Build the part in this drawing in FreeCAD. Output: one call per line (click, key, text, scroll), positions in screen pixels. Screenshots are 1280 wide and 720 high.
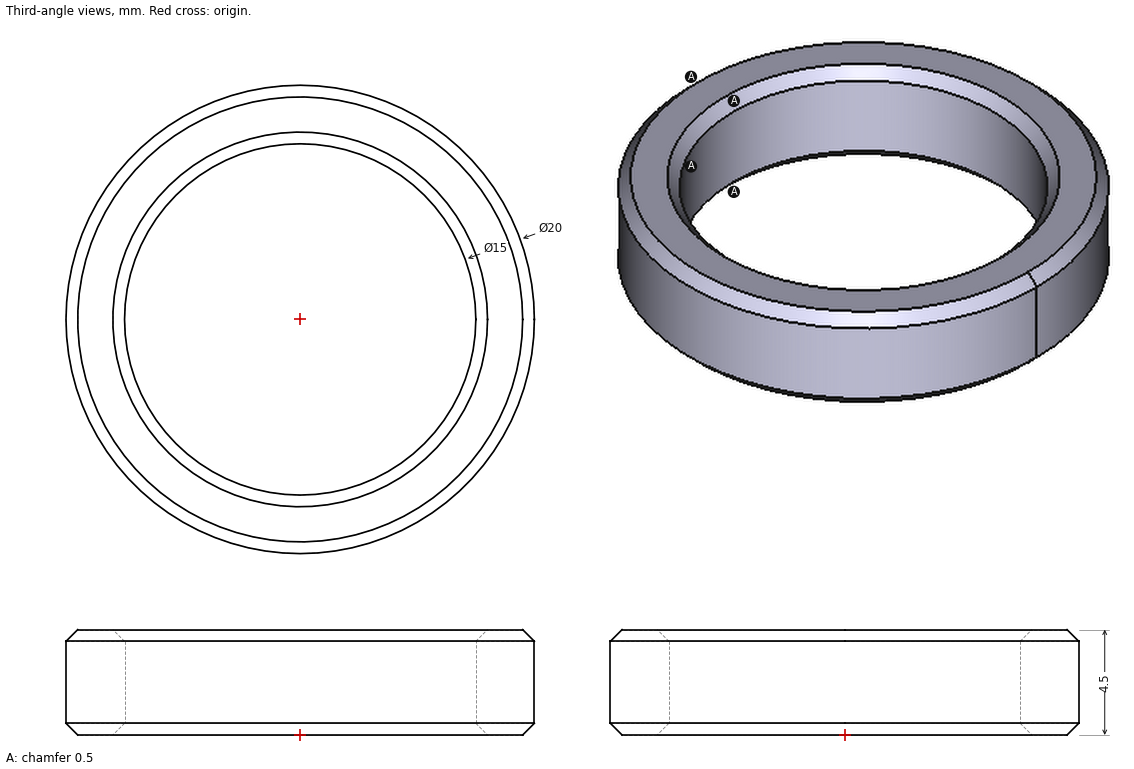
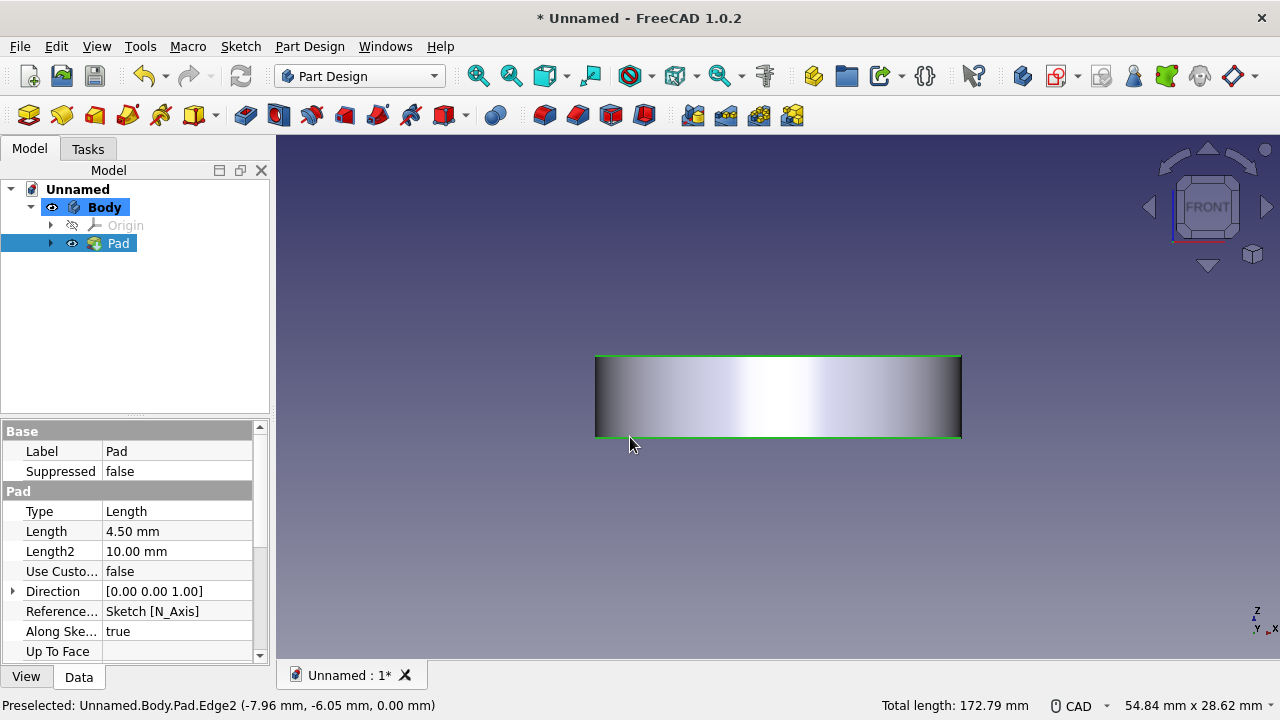
key(3)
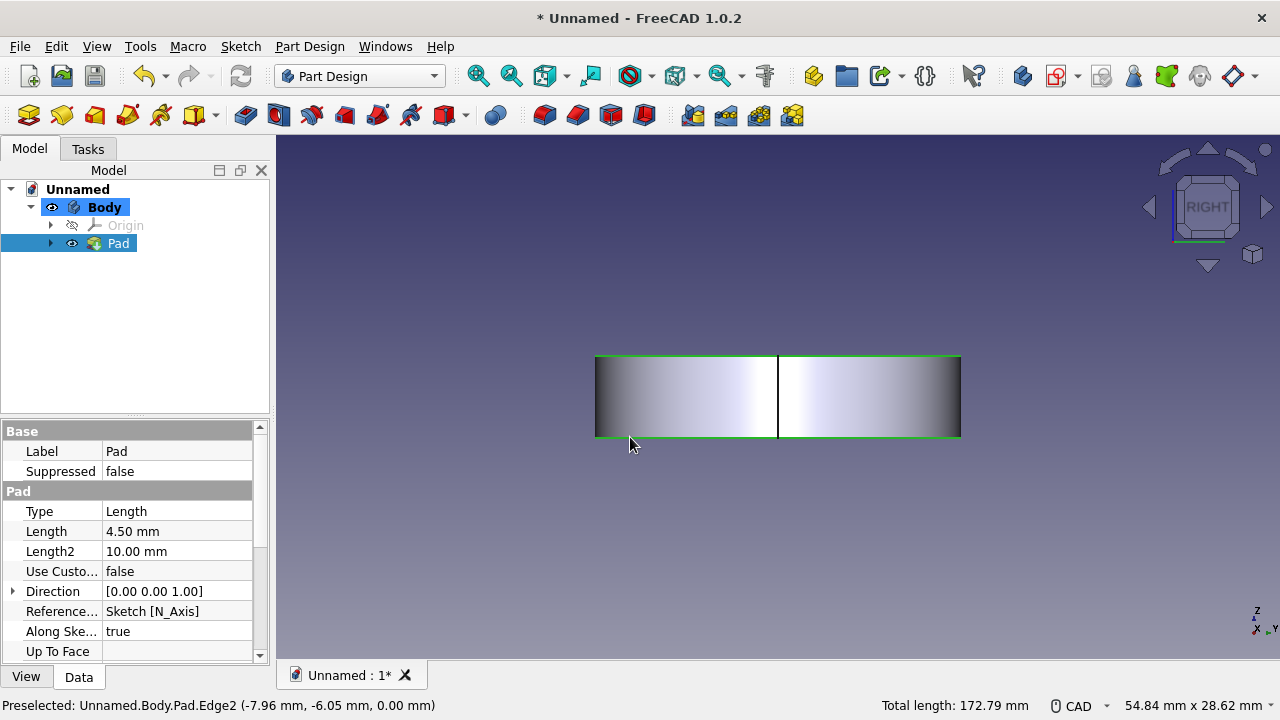
click(479, 76)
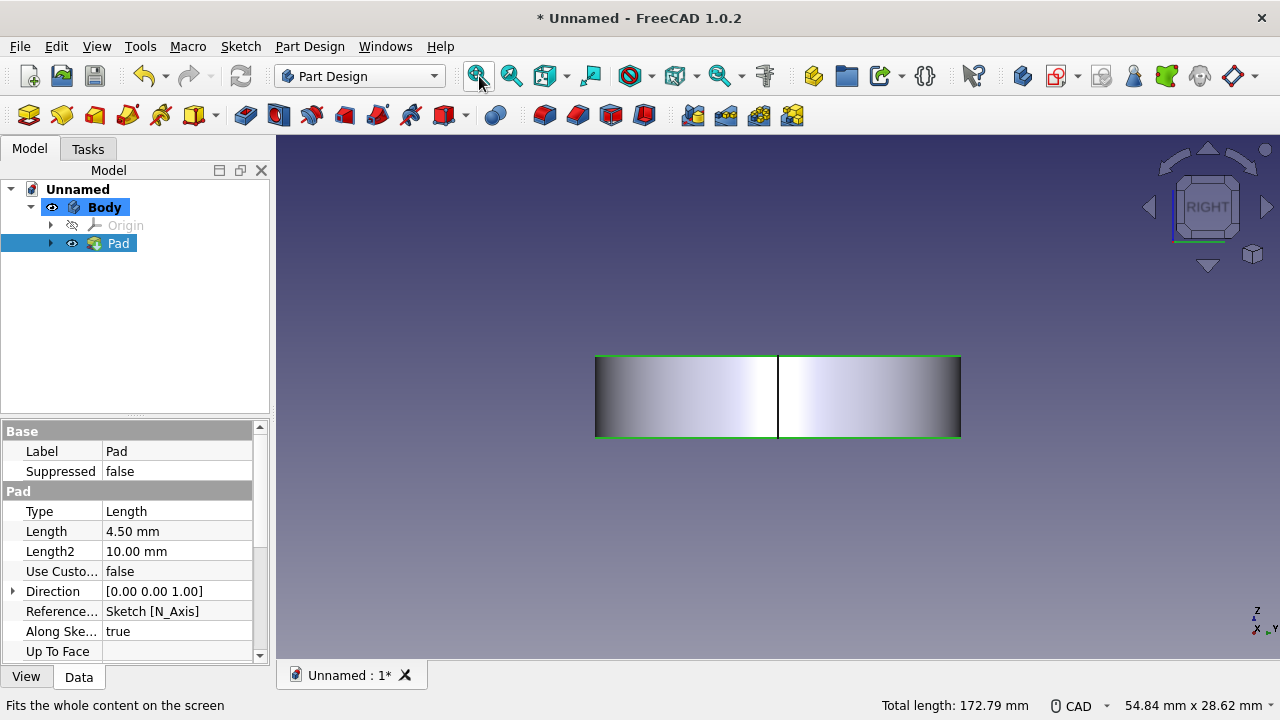
key(5)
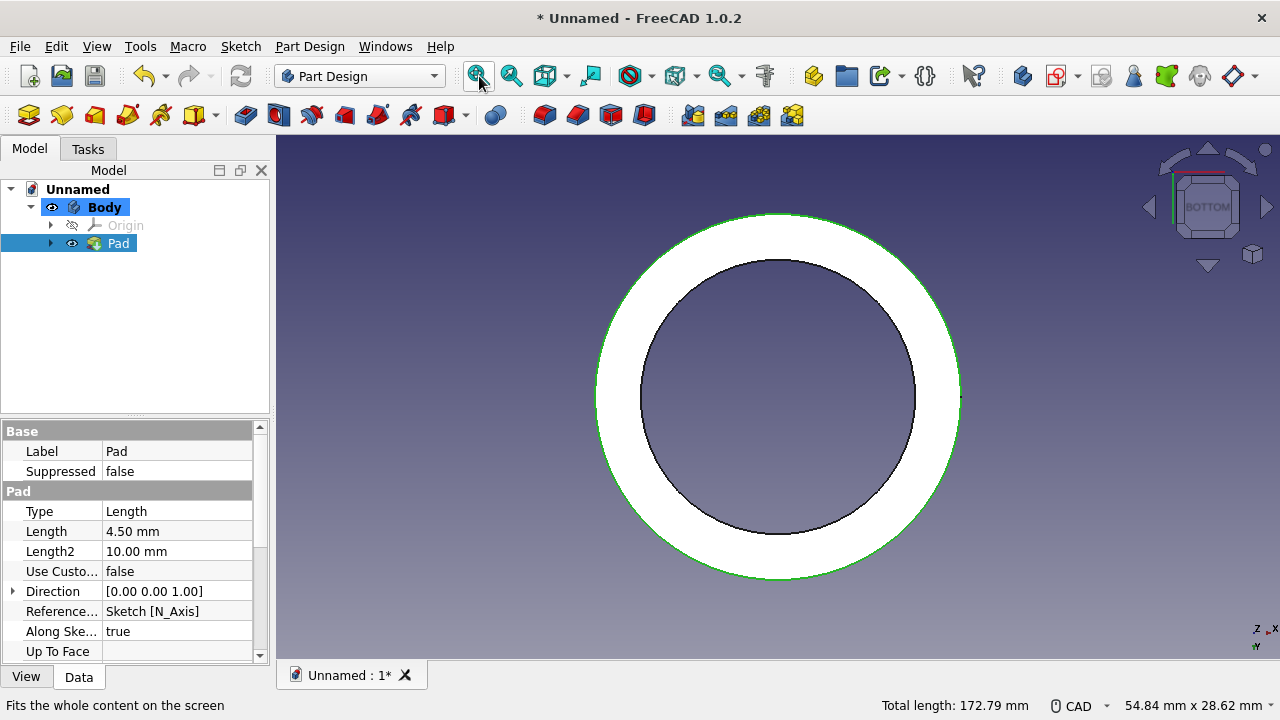
click(667, 477, ctrl)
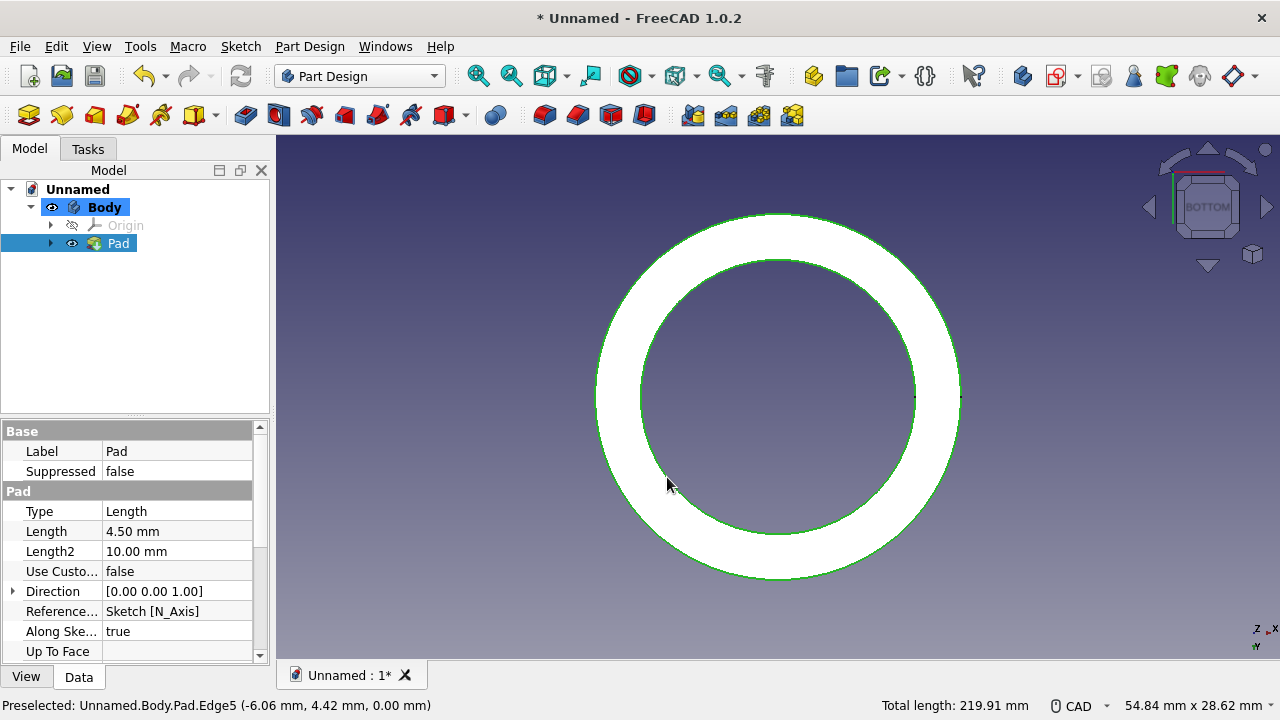
click(578, 116)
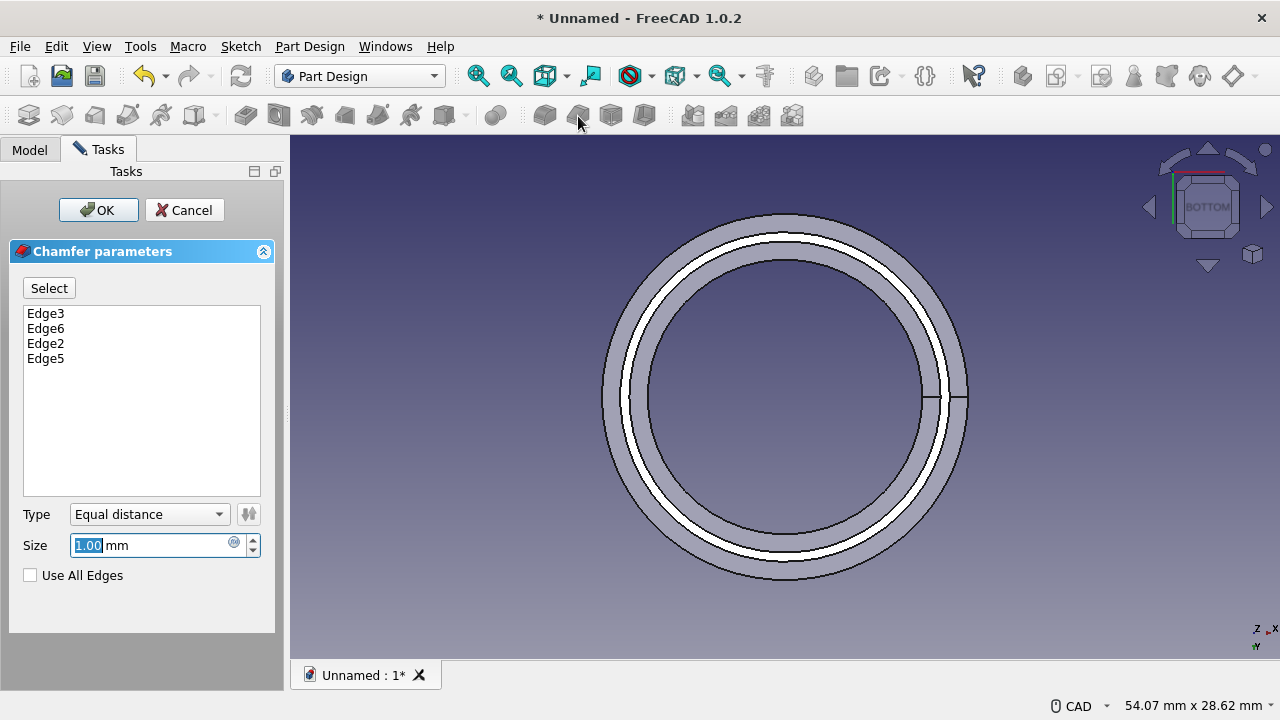
text(0.5)
key(Tab)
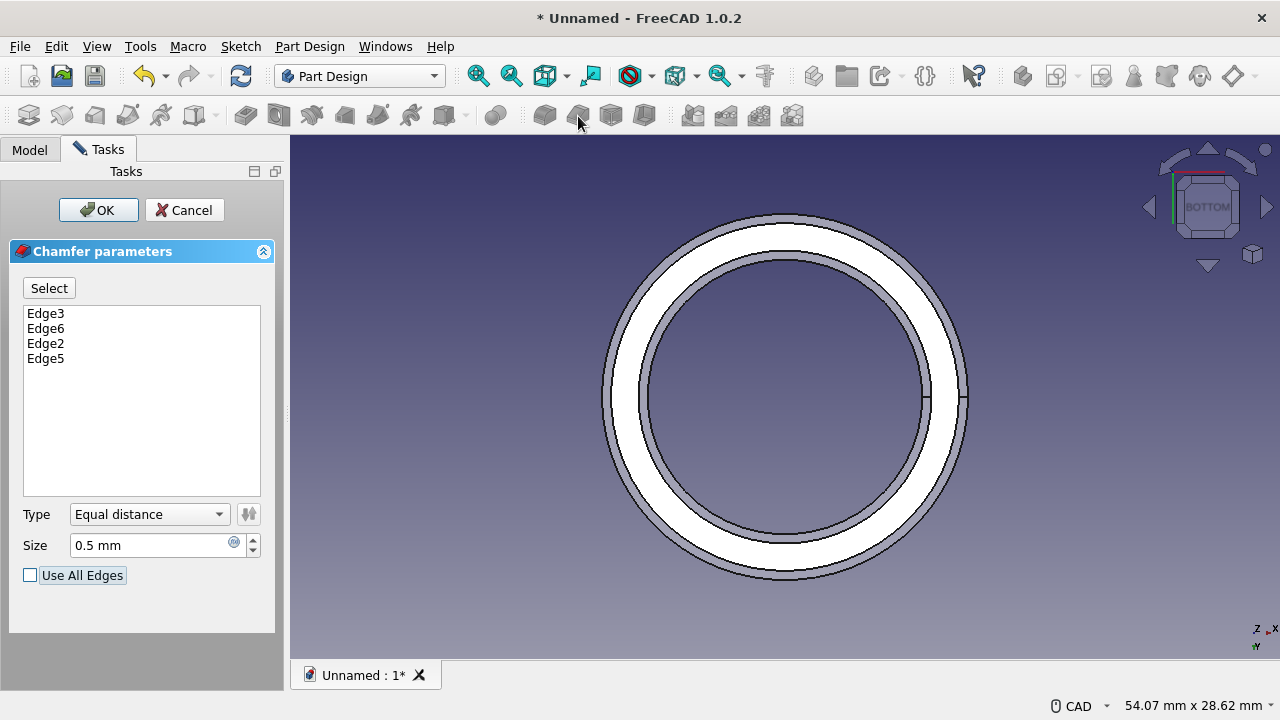
click(99, 210)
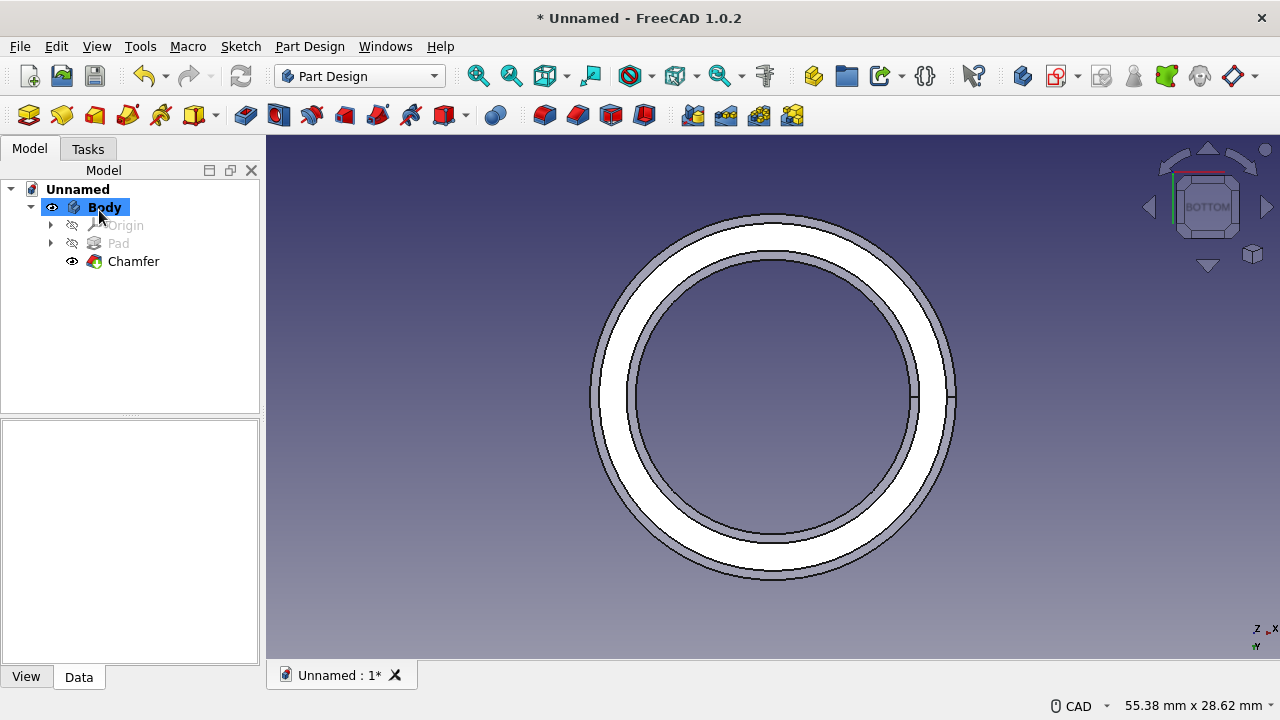
key(0)